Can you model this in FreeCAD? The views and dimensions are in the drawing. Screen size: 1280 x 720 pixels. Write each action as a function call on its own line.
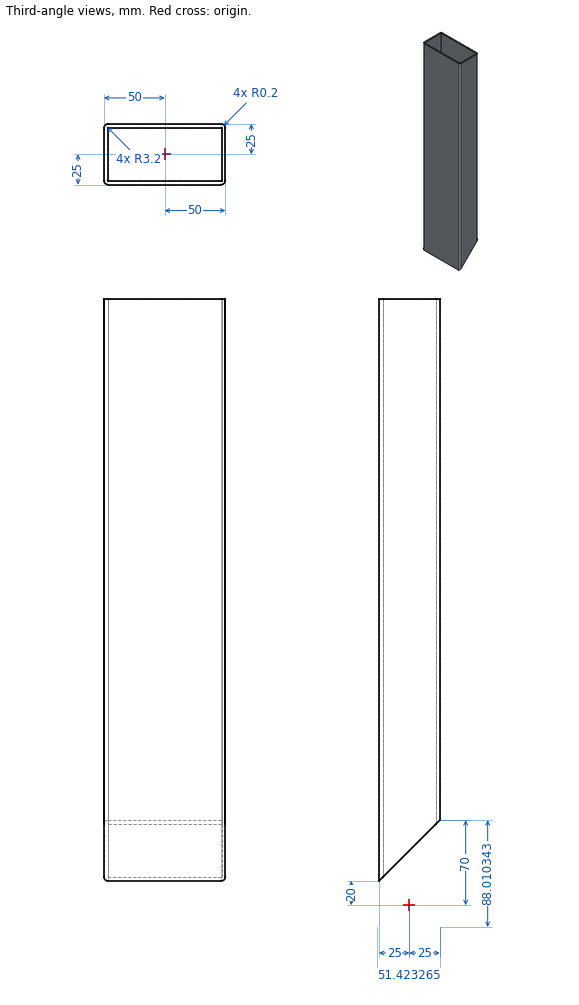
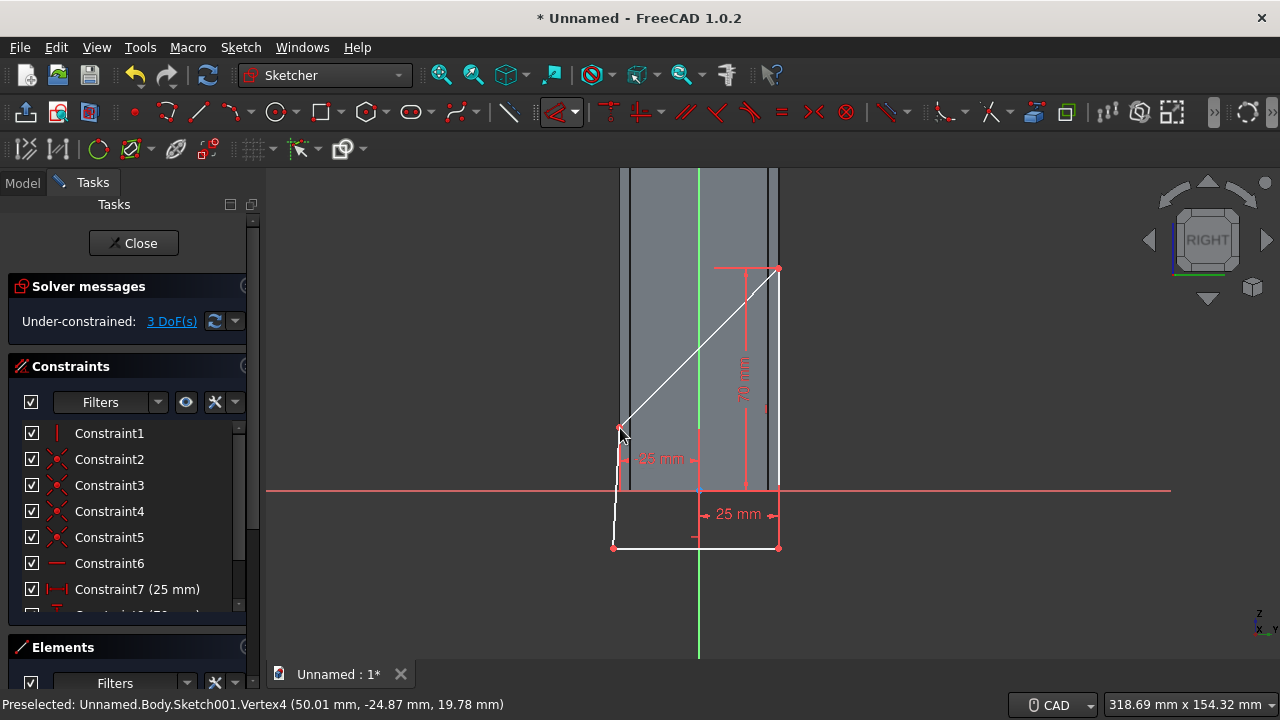
click(620, 428)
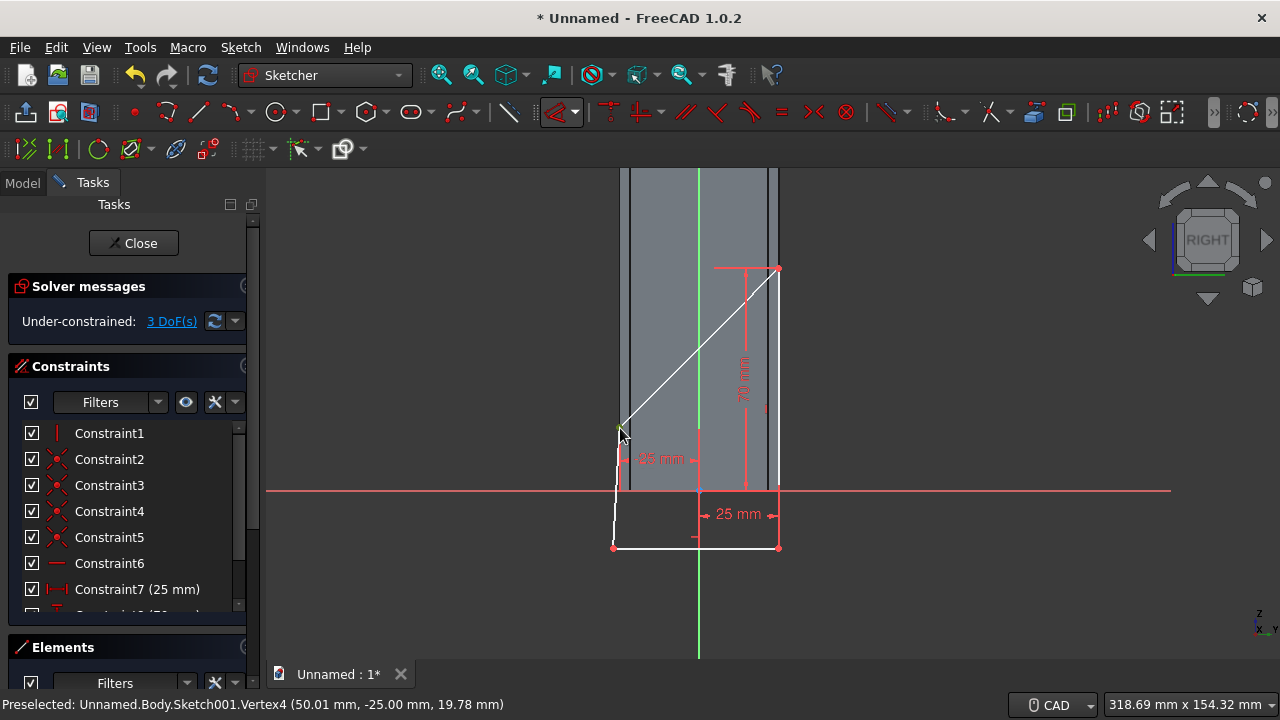
click(578, 112)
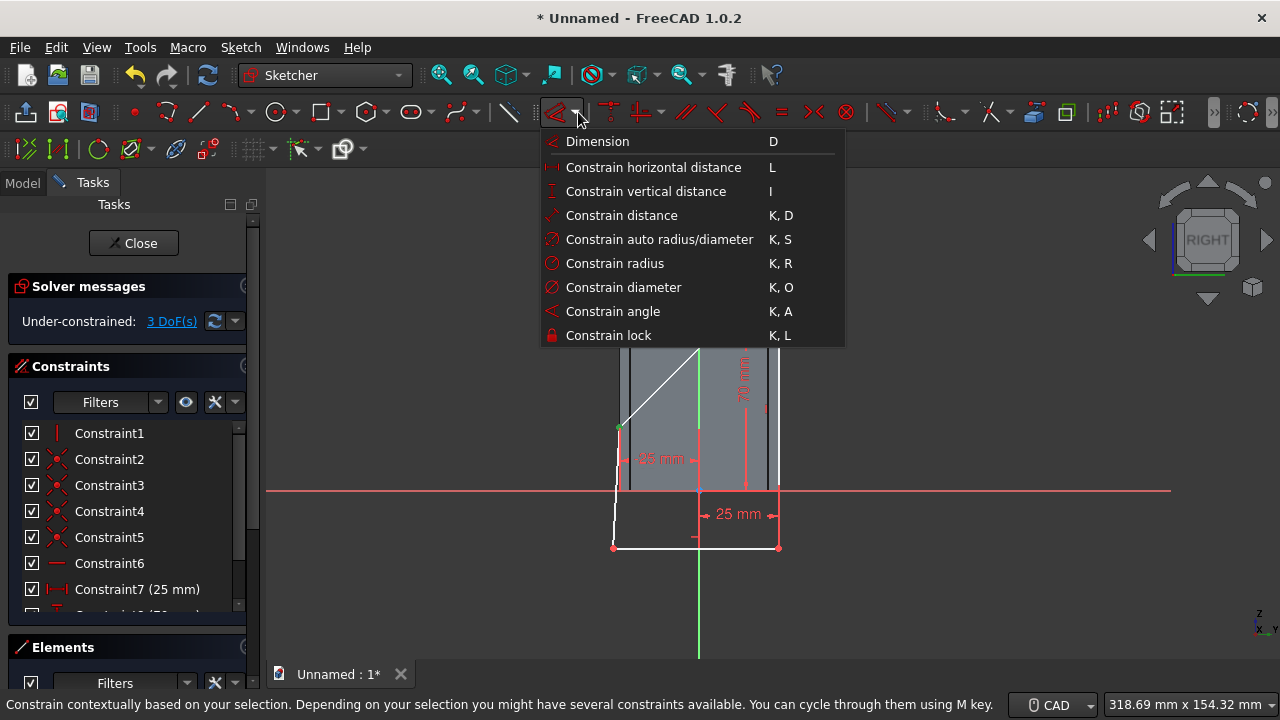
click(693, 191)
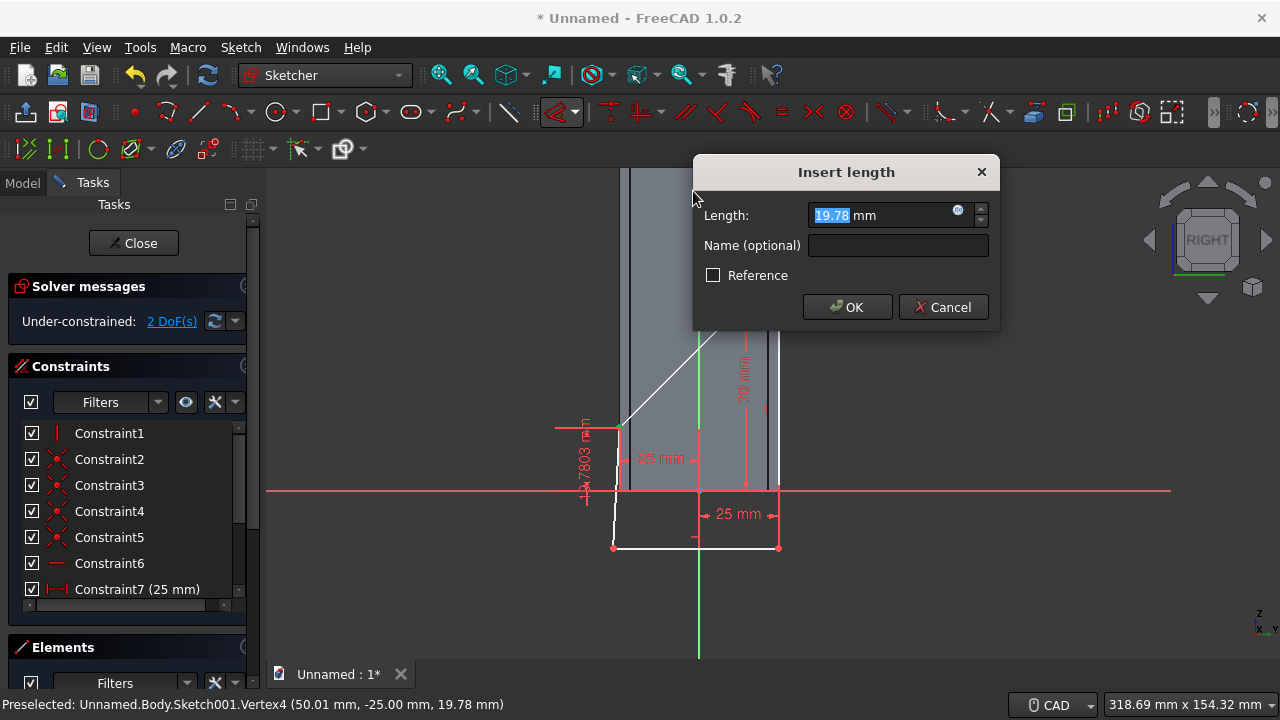
text(20)
key(Return)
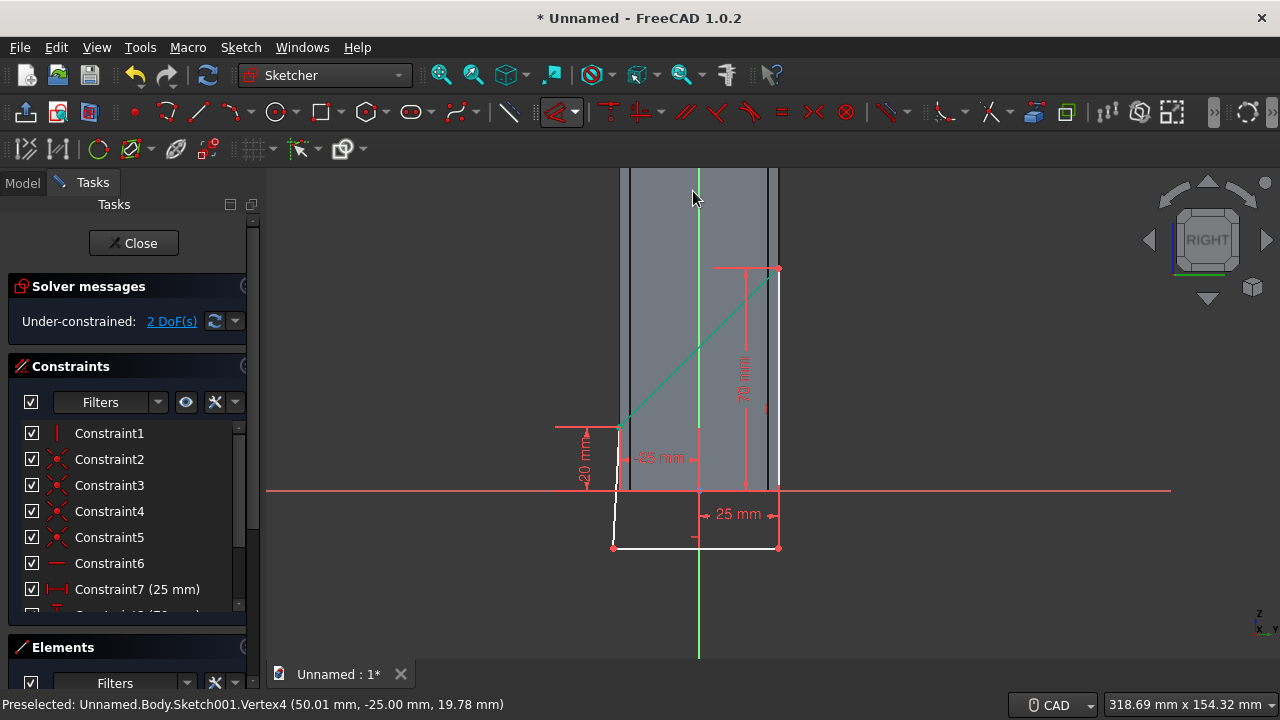
click(779, 465)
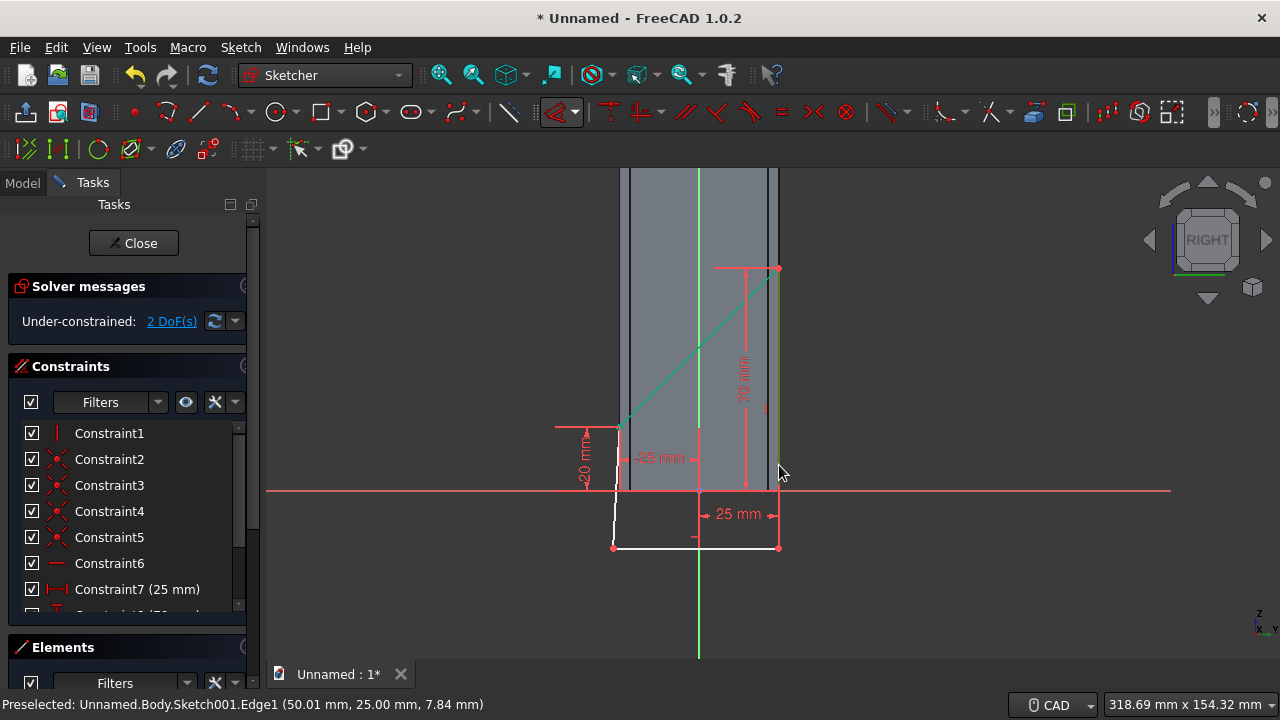
key(i)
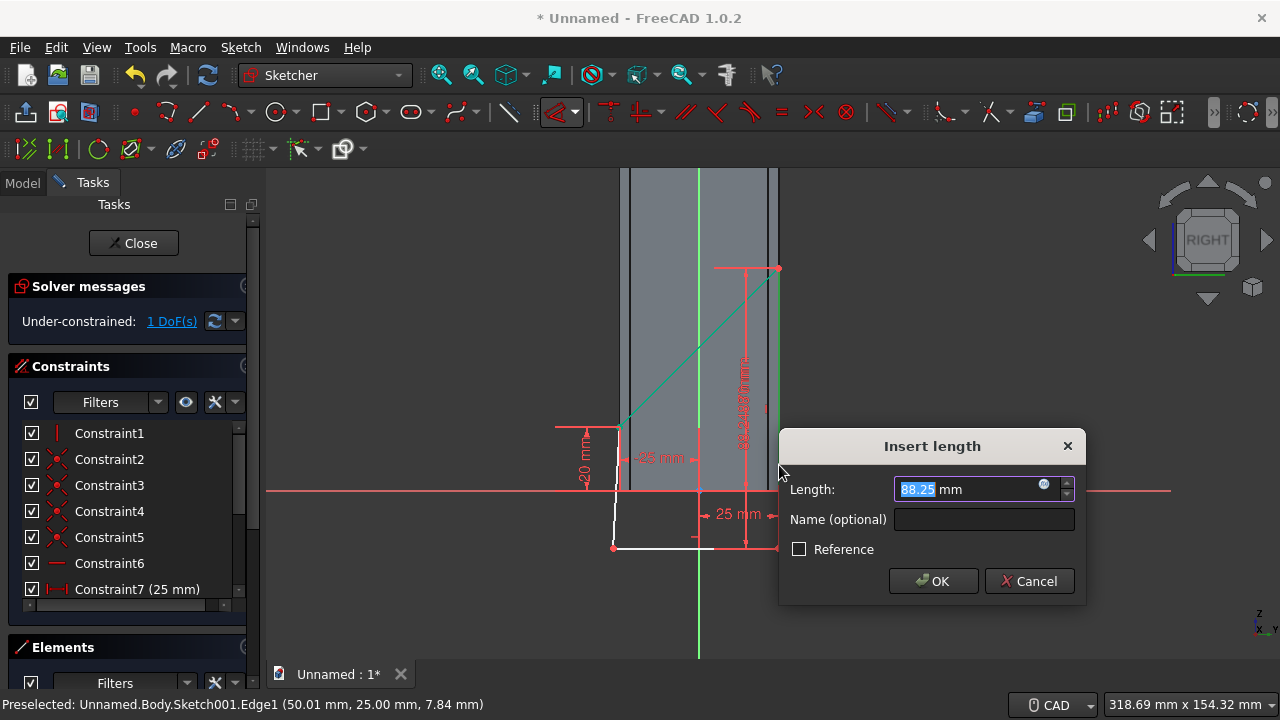
text(88.010343)
key(Return)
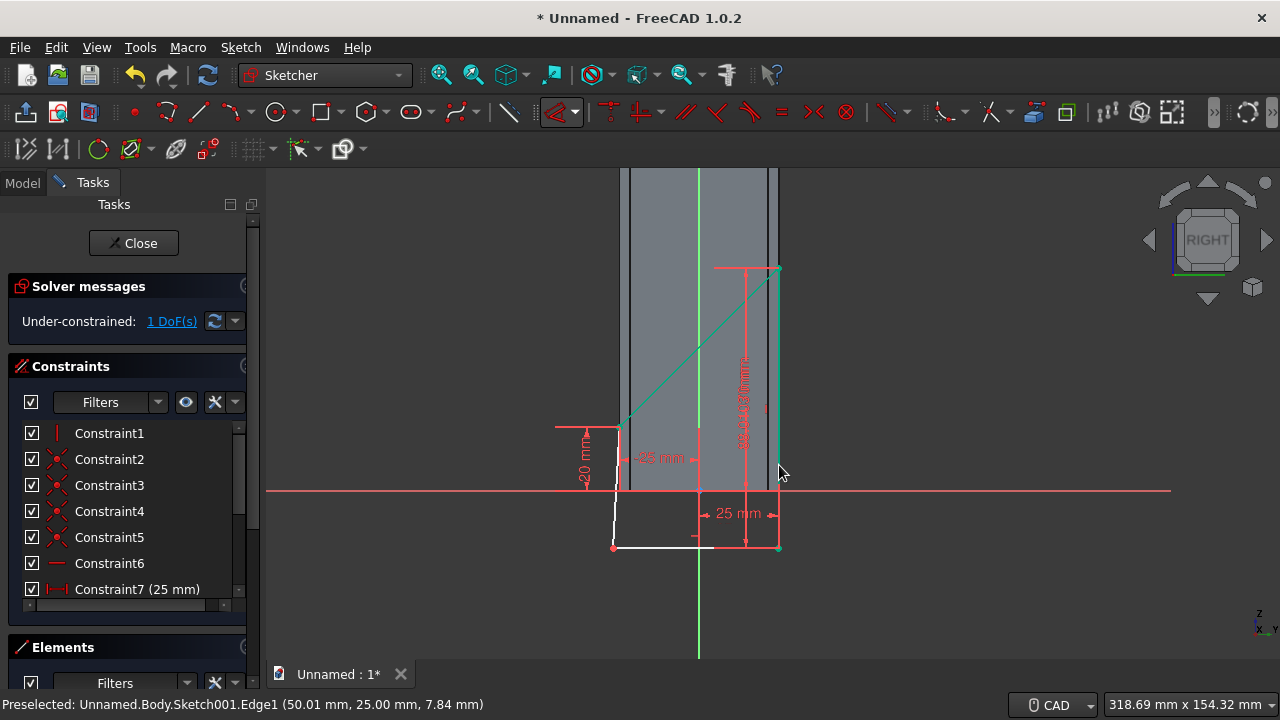
click(663, 548)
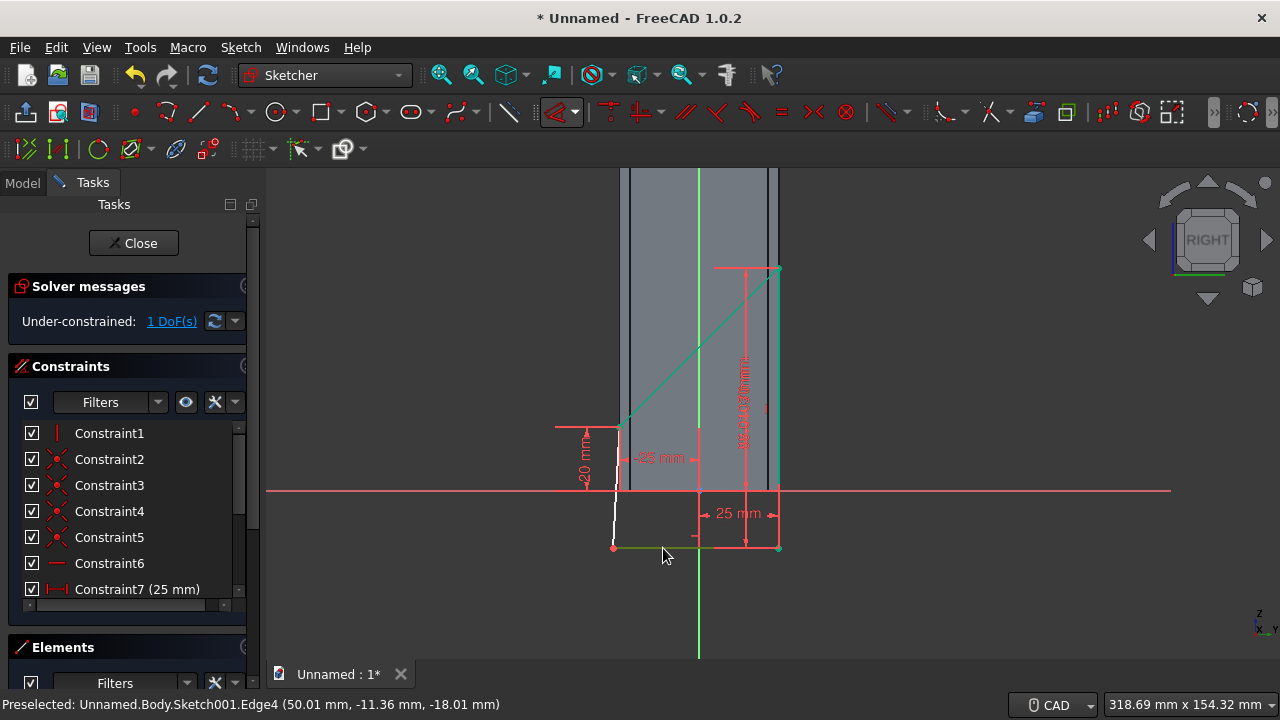
key(l)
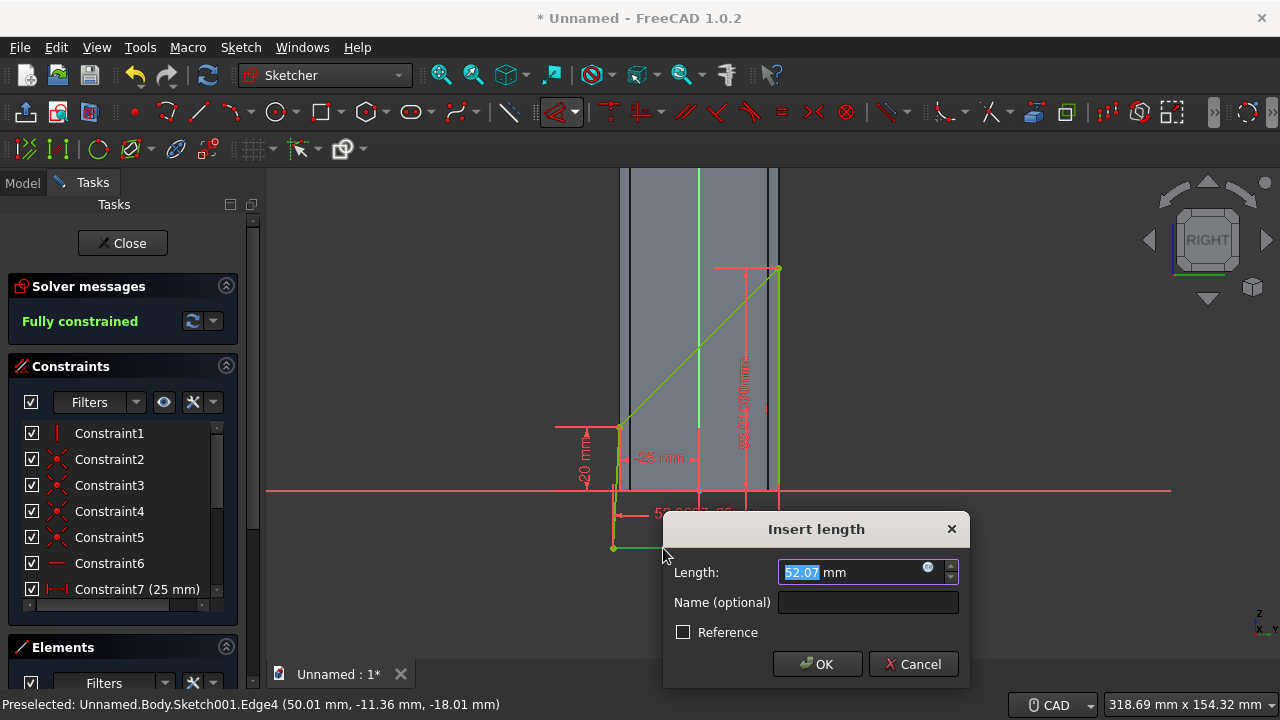
text(51.423265)
key(Return)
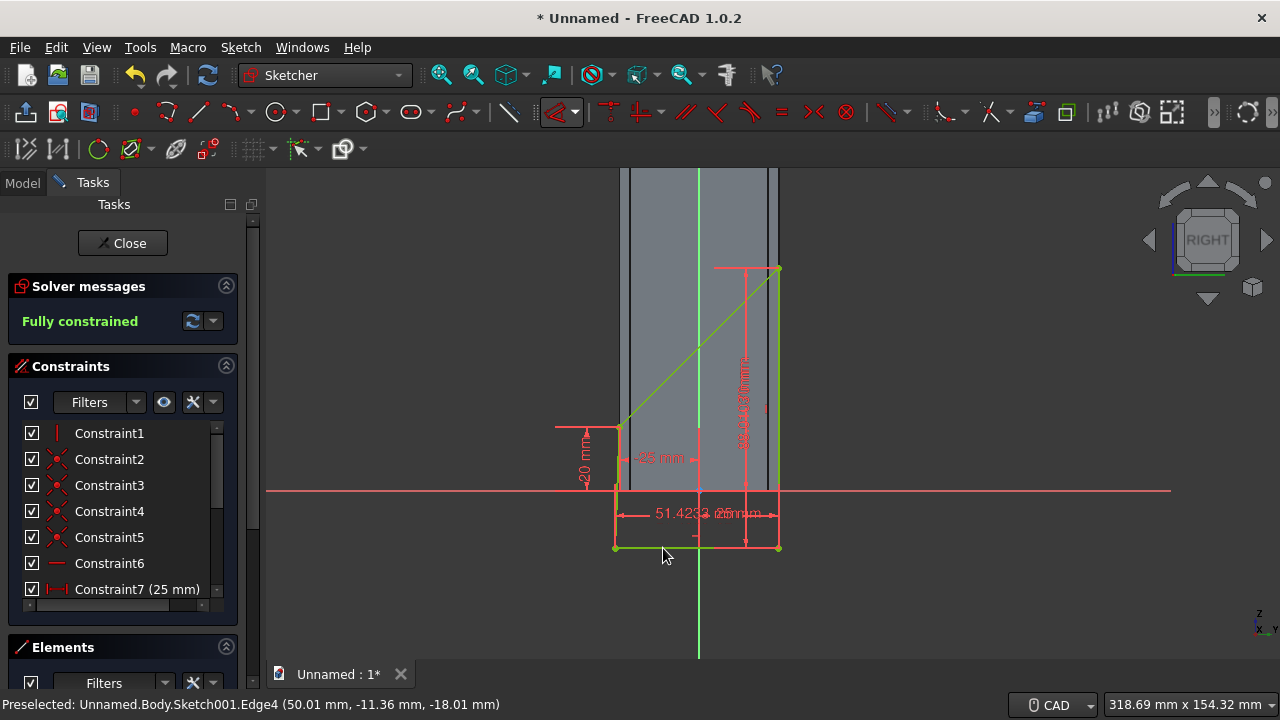
click(123, 243)